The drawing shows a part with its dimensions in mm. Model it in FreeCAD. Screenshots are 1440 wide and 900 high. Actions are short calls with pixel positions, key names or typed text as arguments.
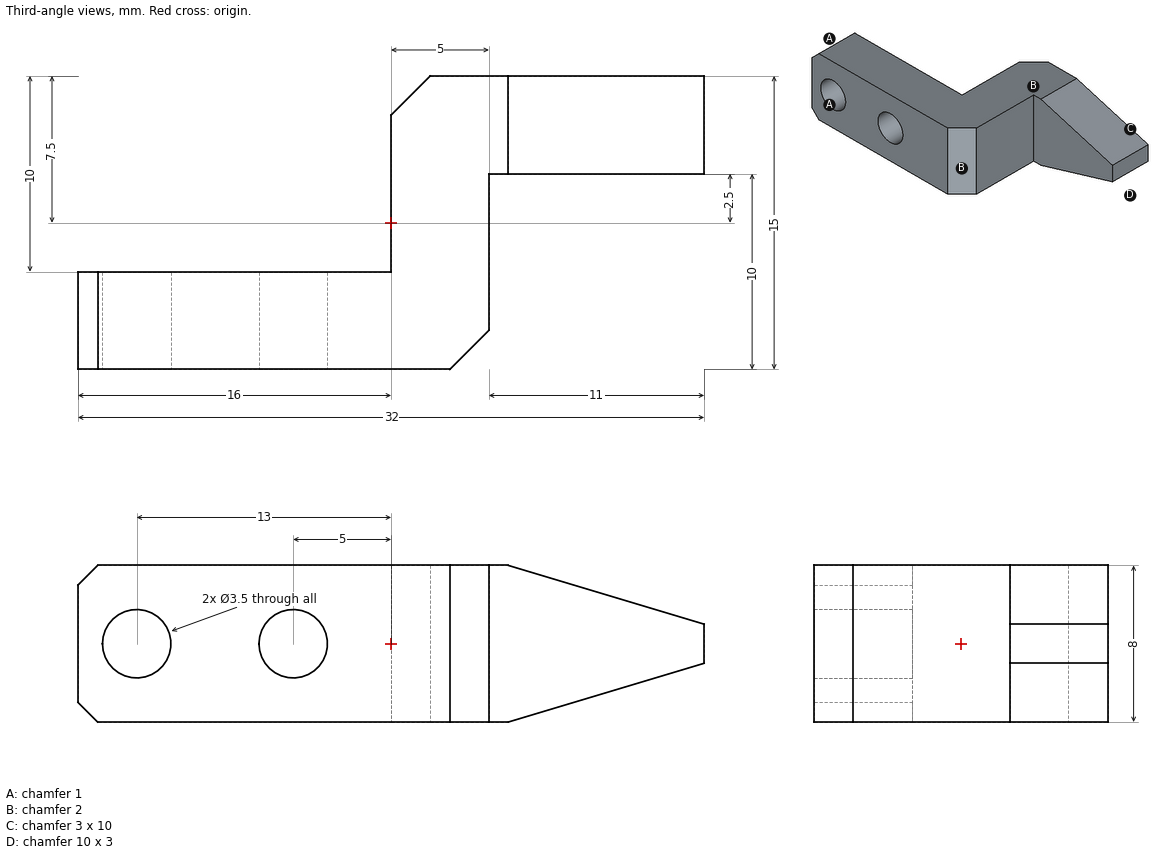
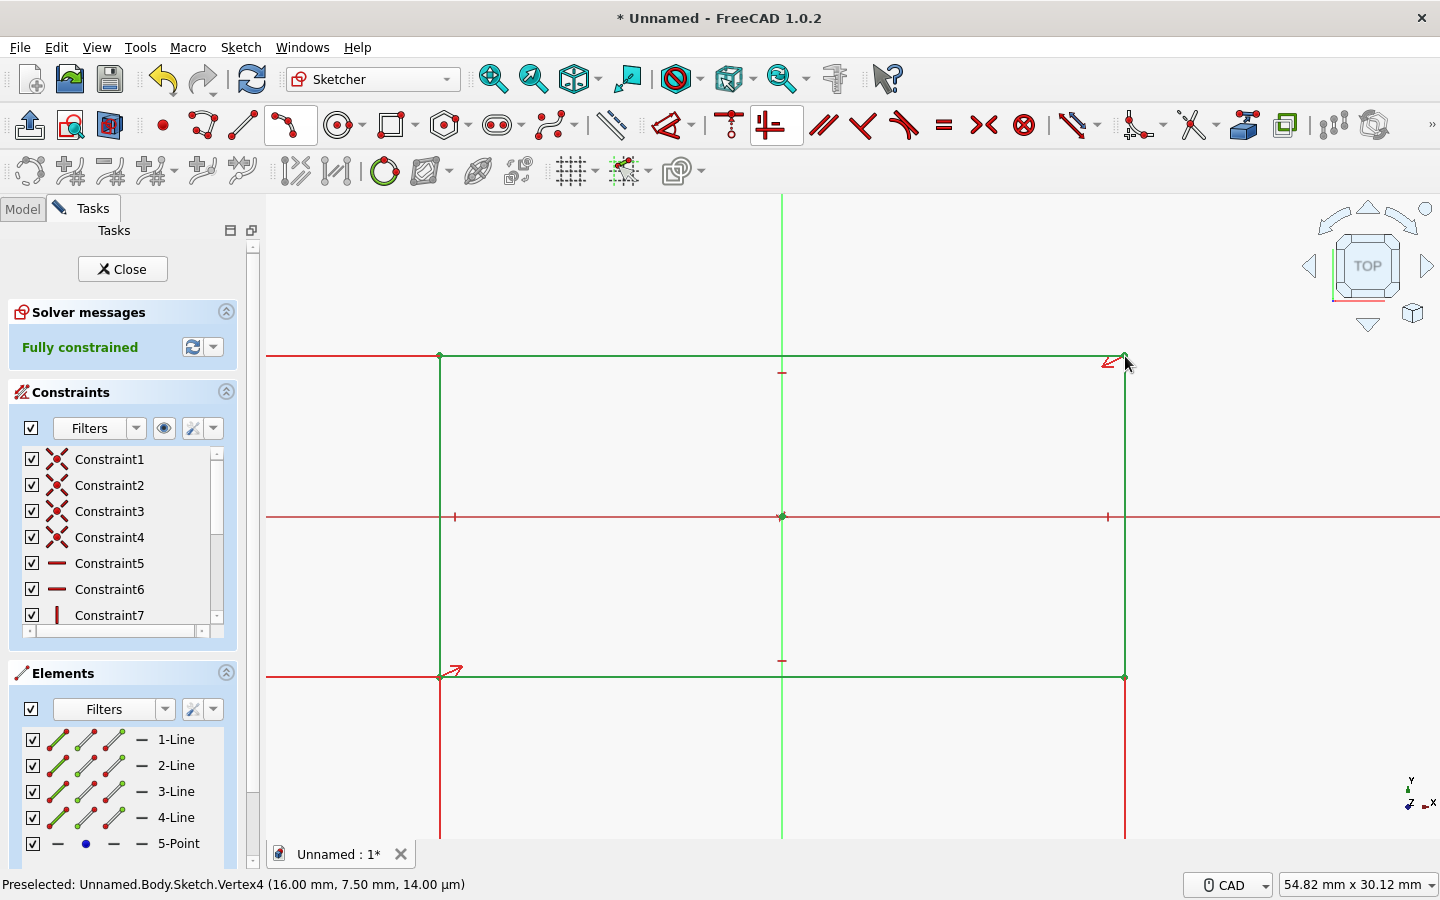
click(123, 269)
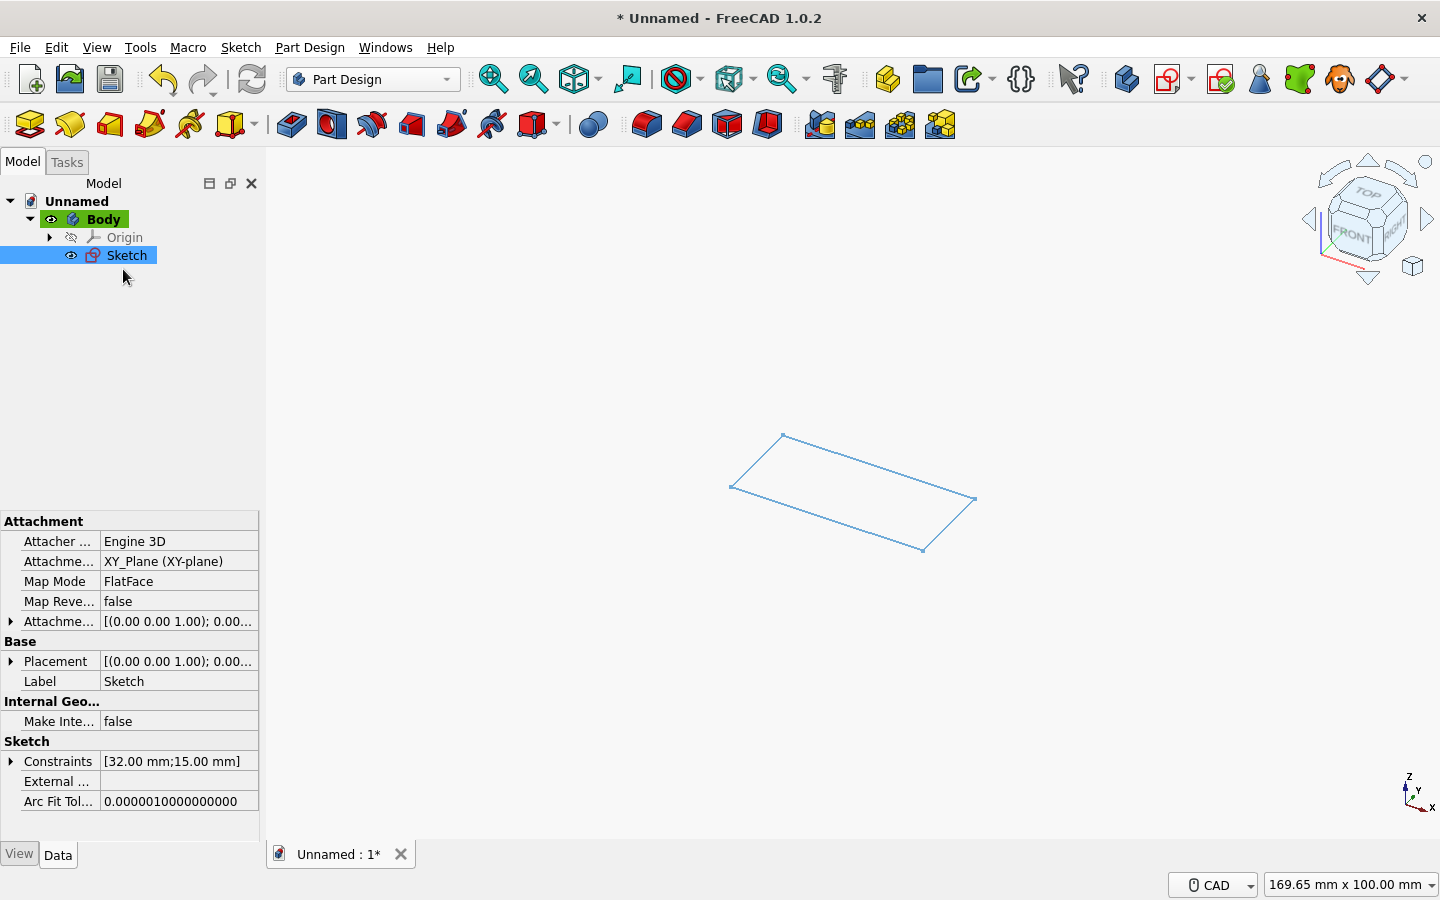
click(30, 124)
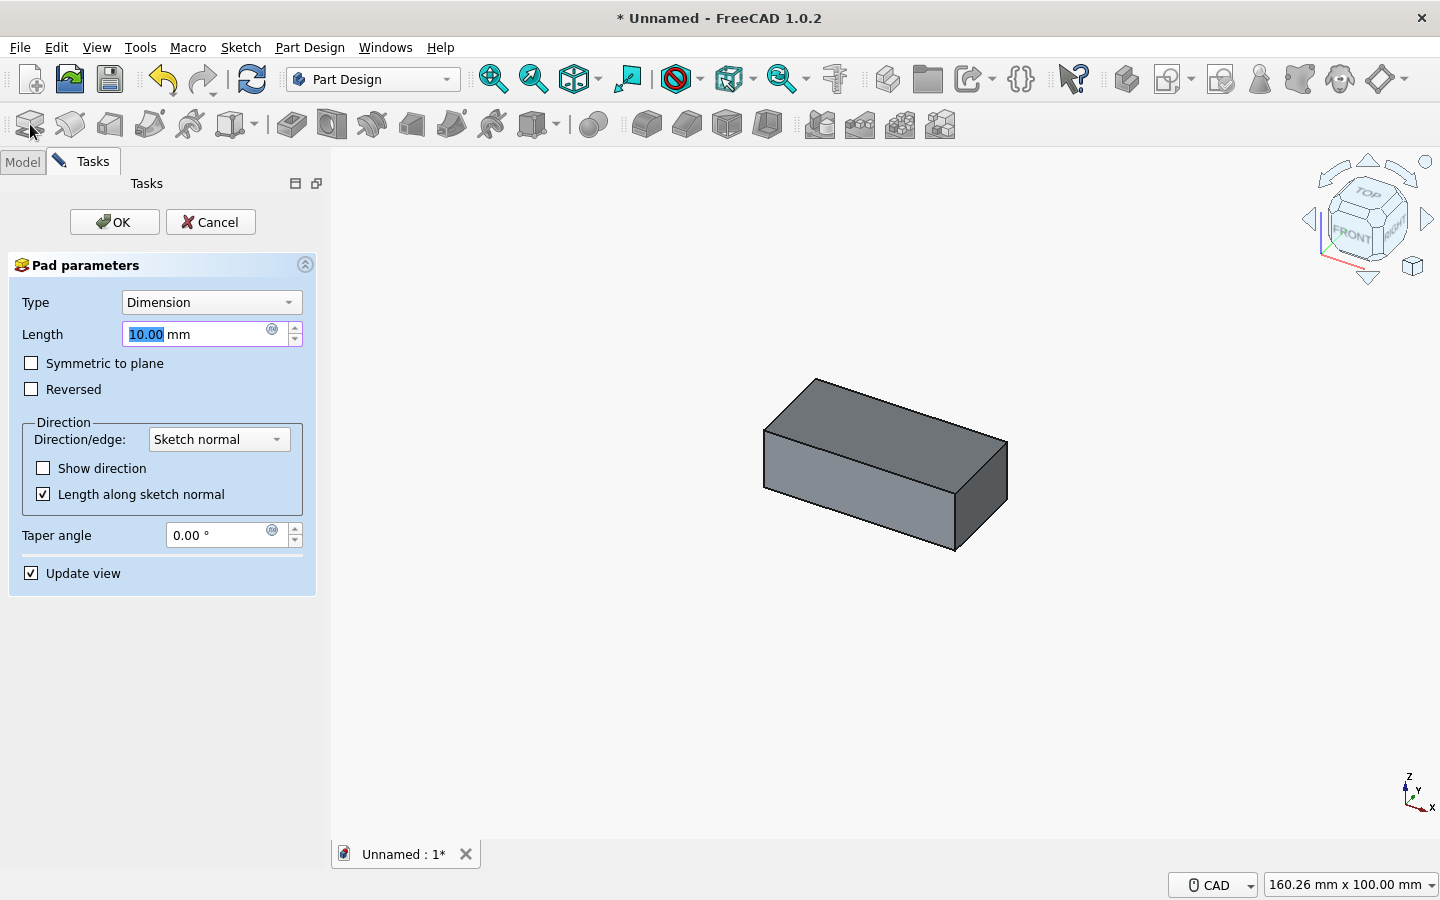
text(8)
key(Tab)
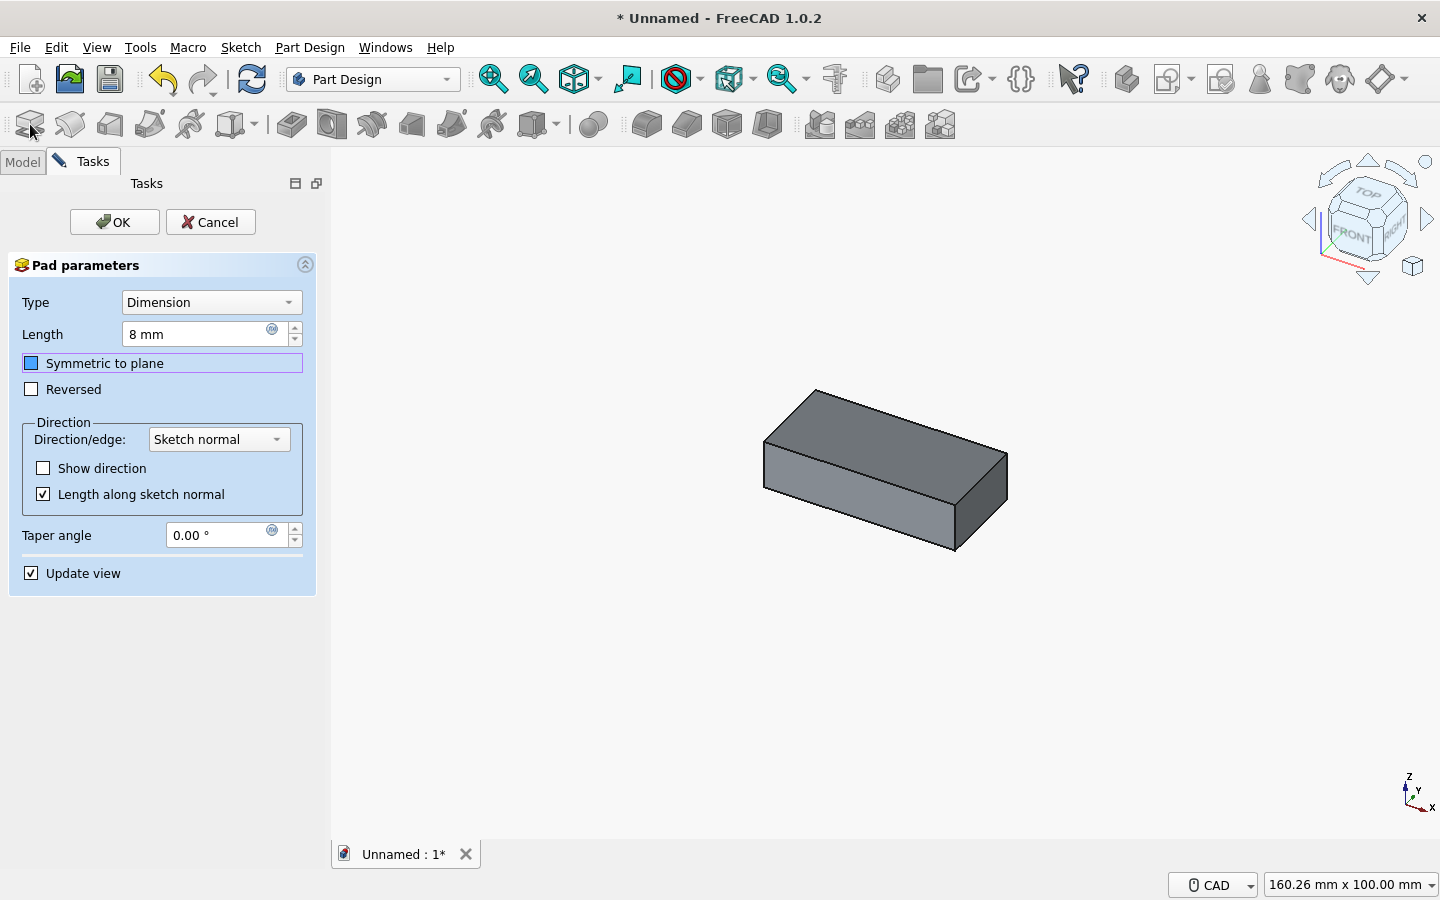
click(30, 363)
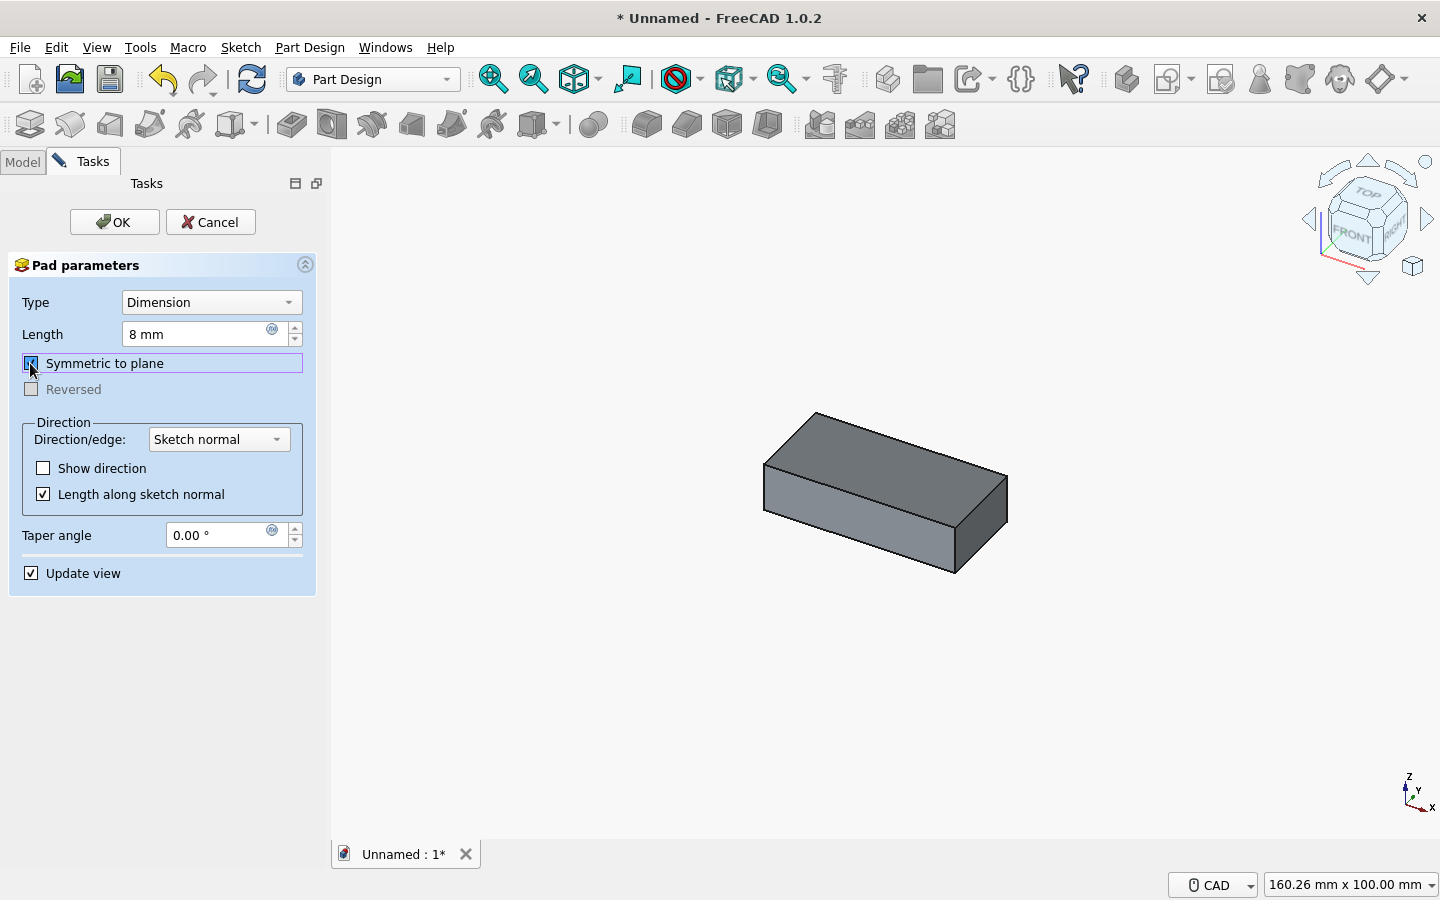
click(115, 222)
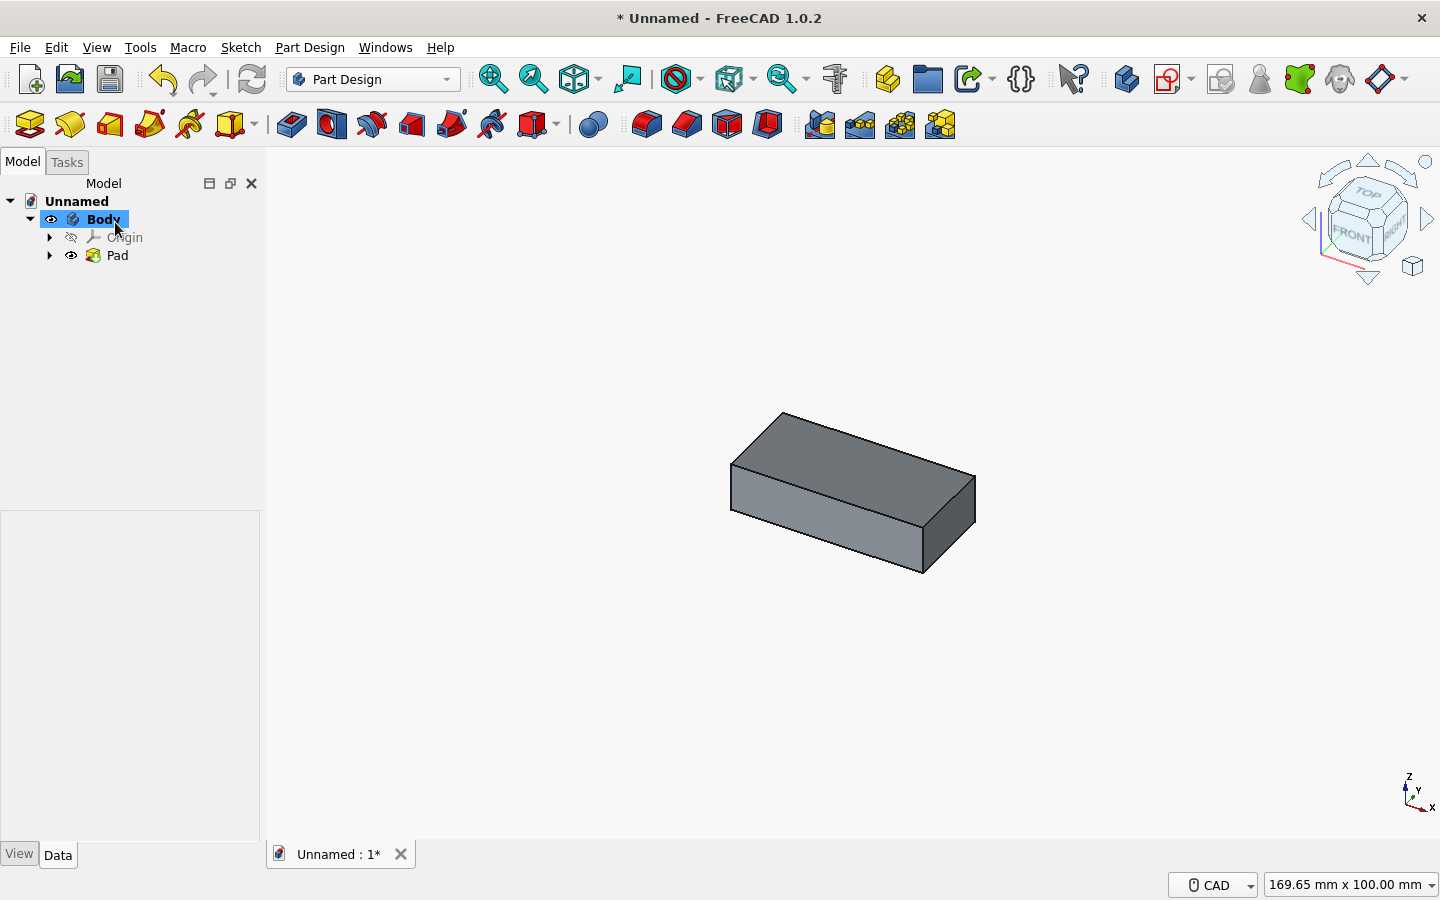
key(v)
key(f)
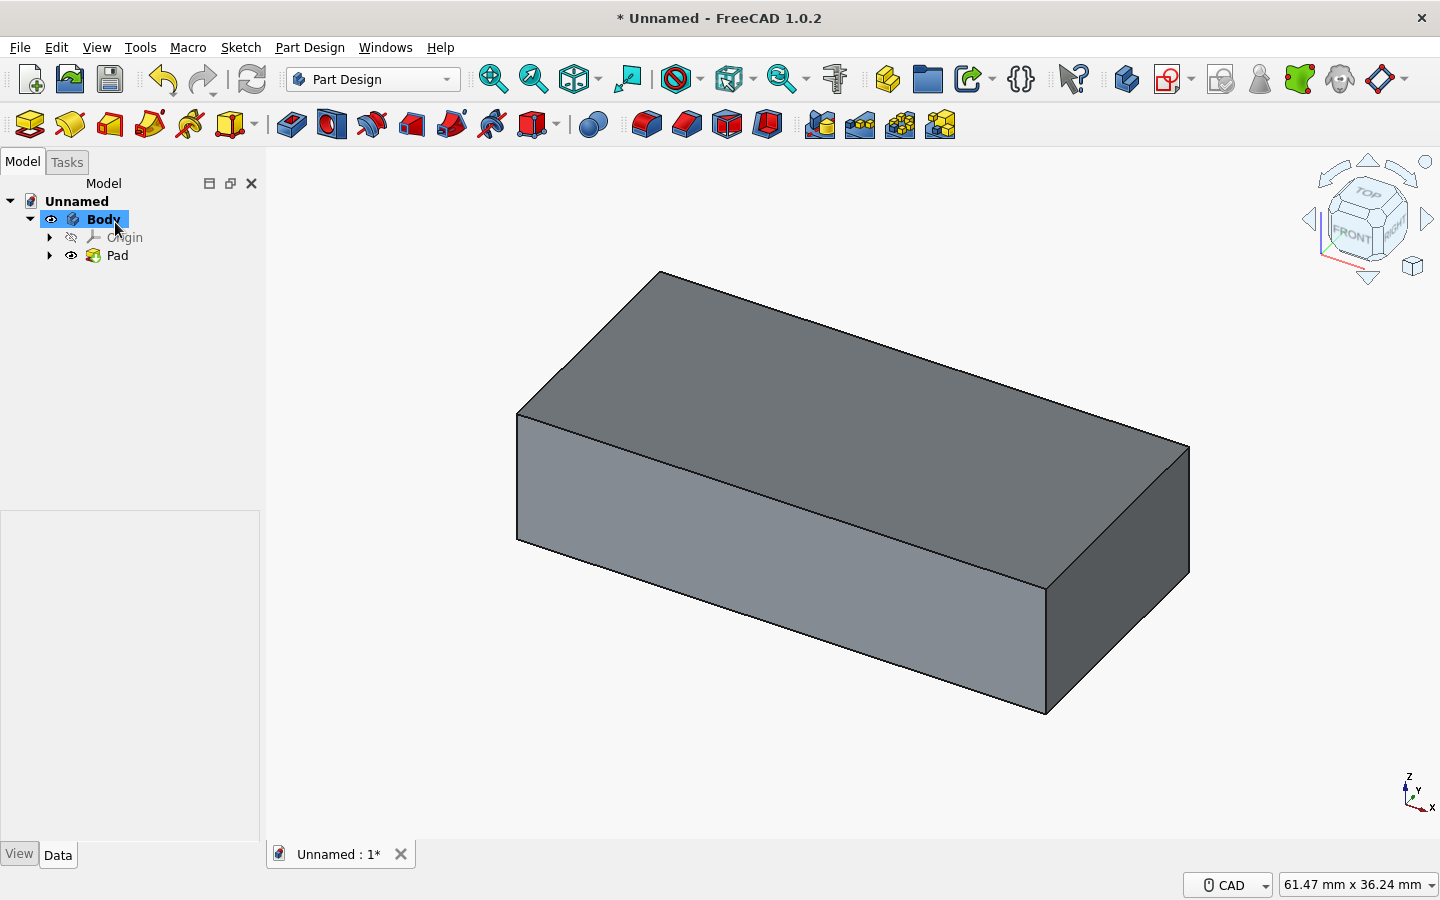
click(929, 454)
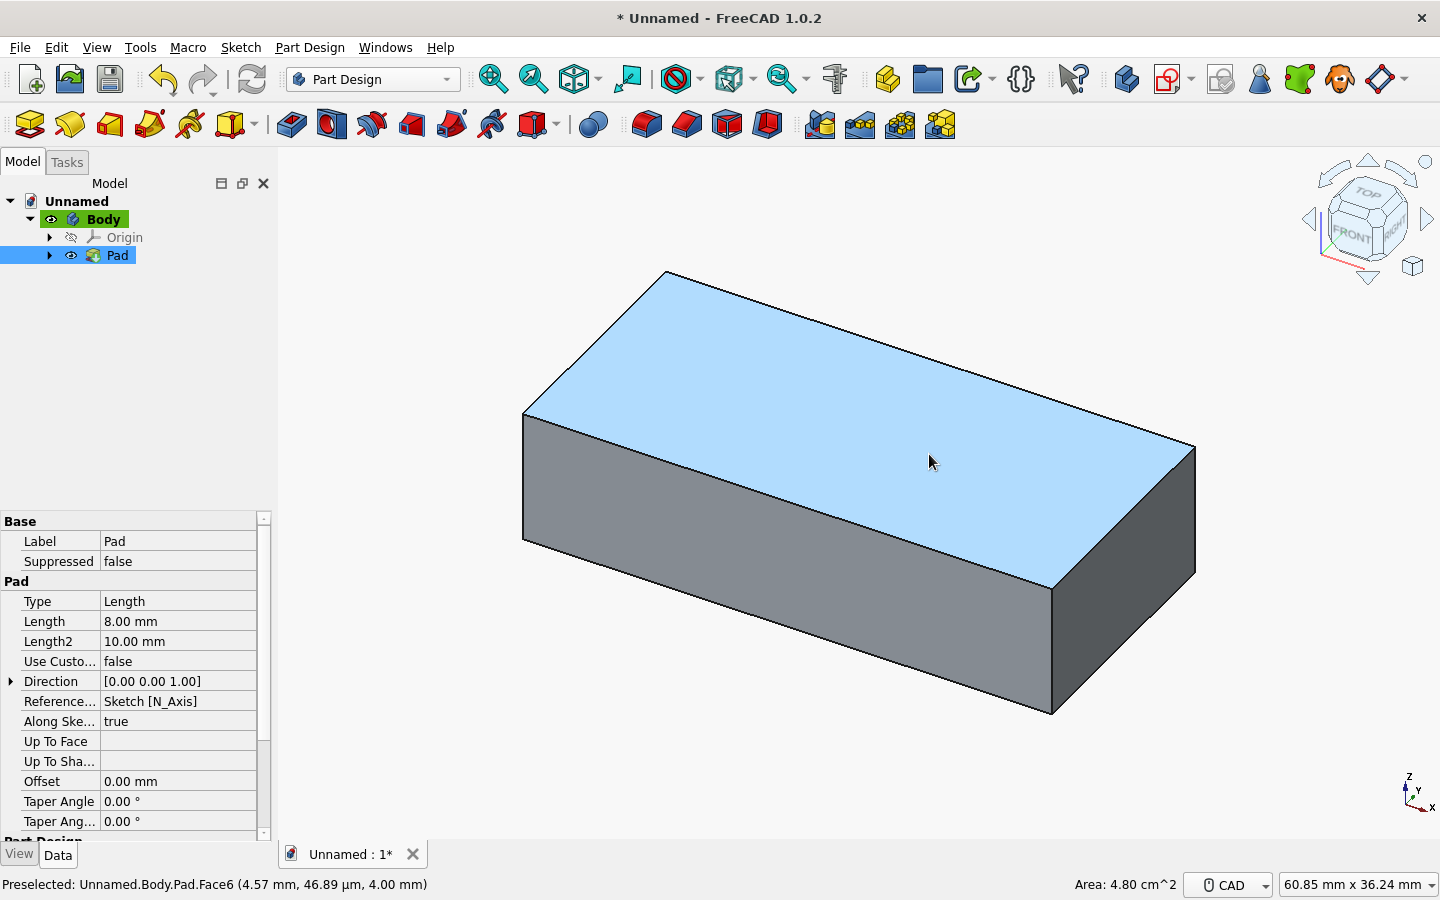
click(1168, 80)